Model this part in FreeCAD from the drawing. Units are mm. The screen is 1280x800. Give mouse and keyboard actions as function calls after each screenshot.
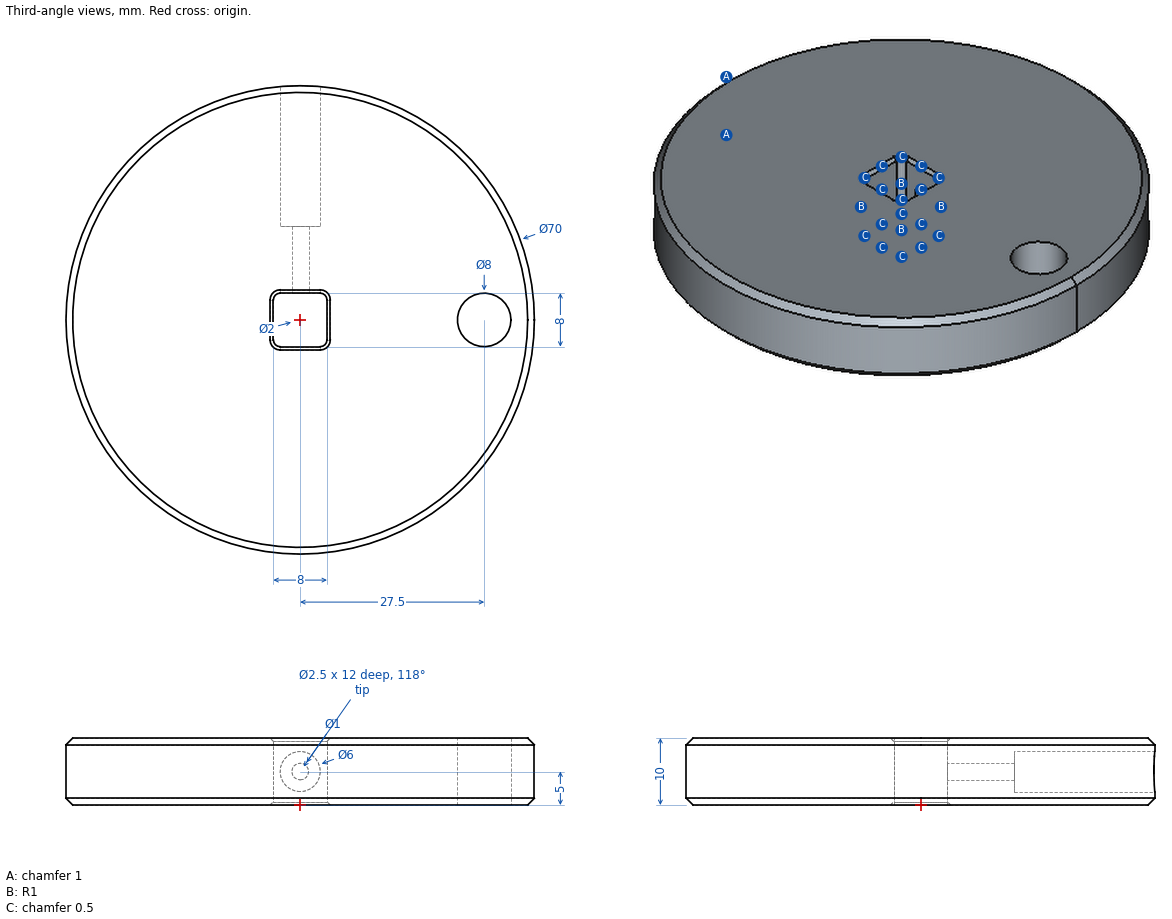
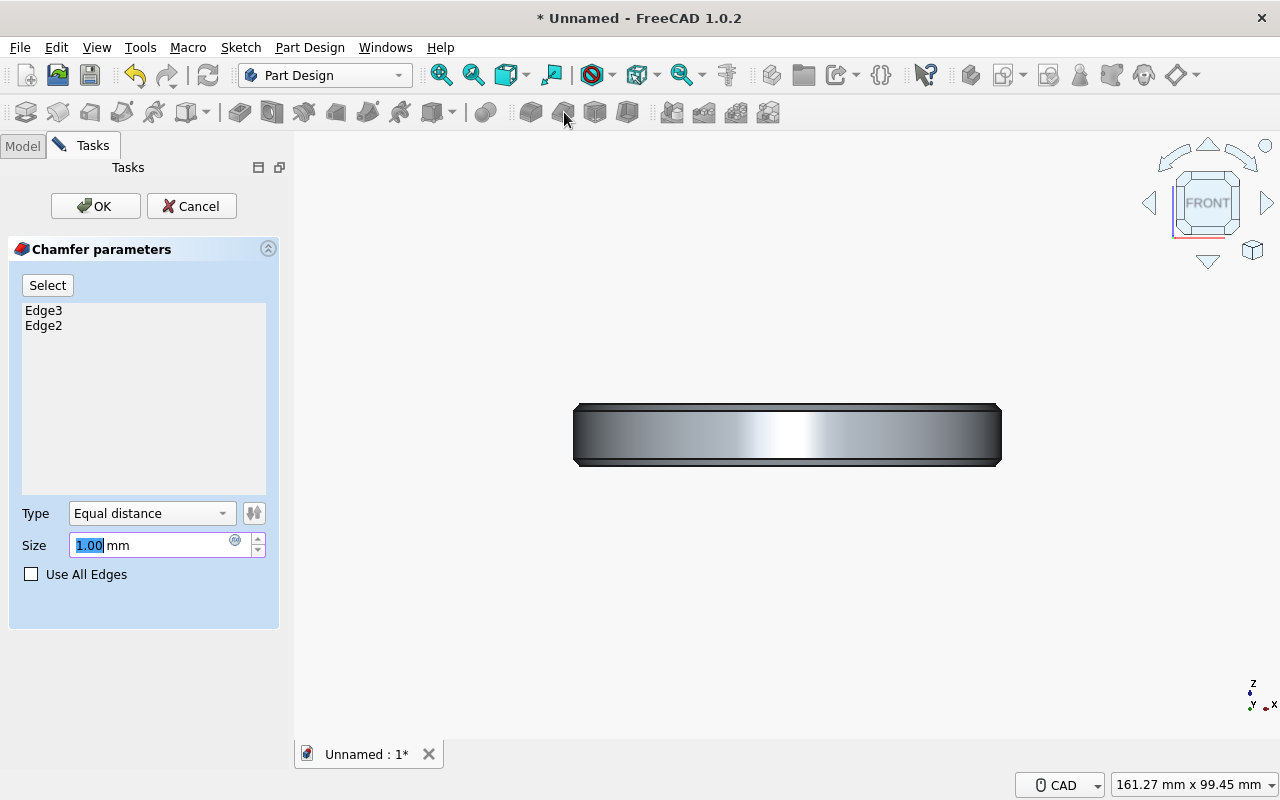
text(1)
key(Tab)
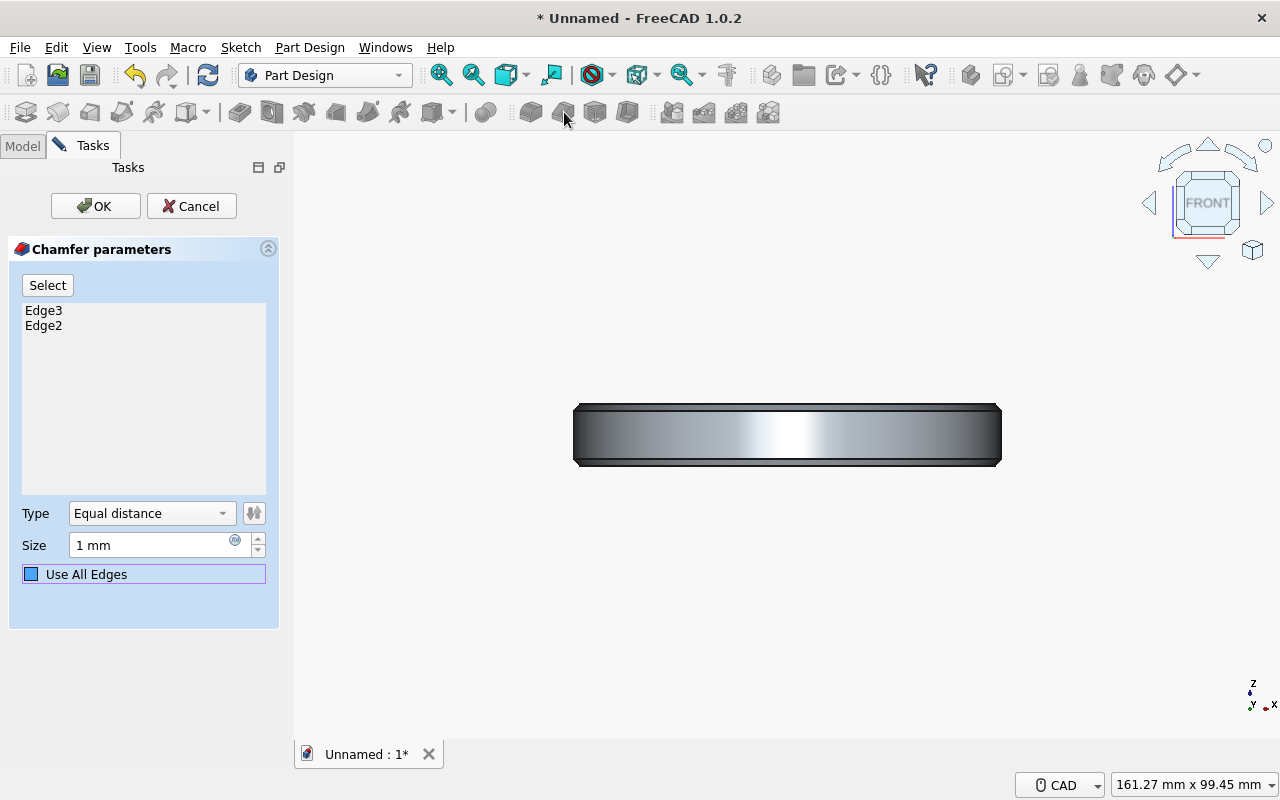
click(96, 206)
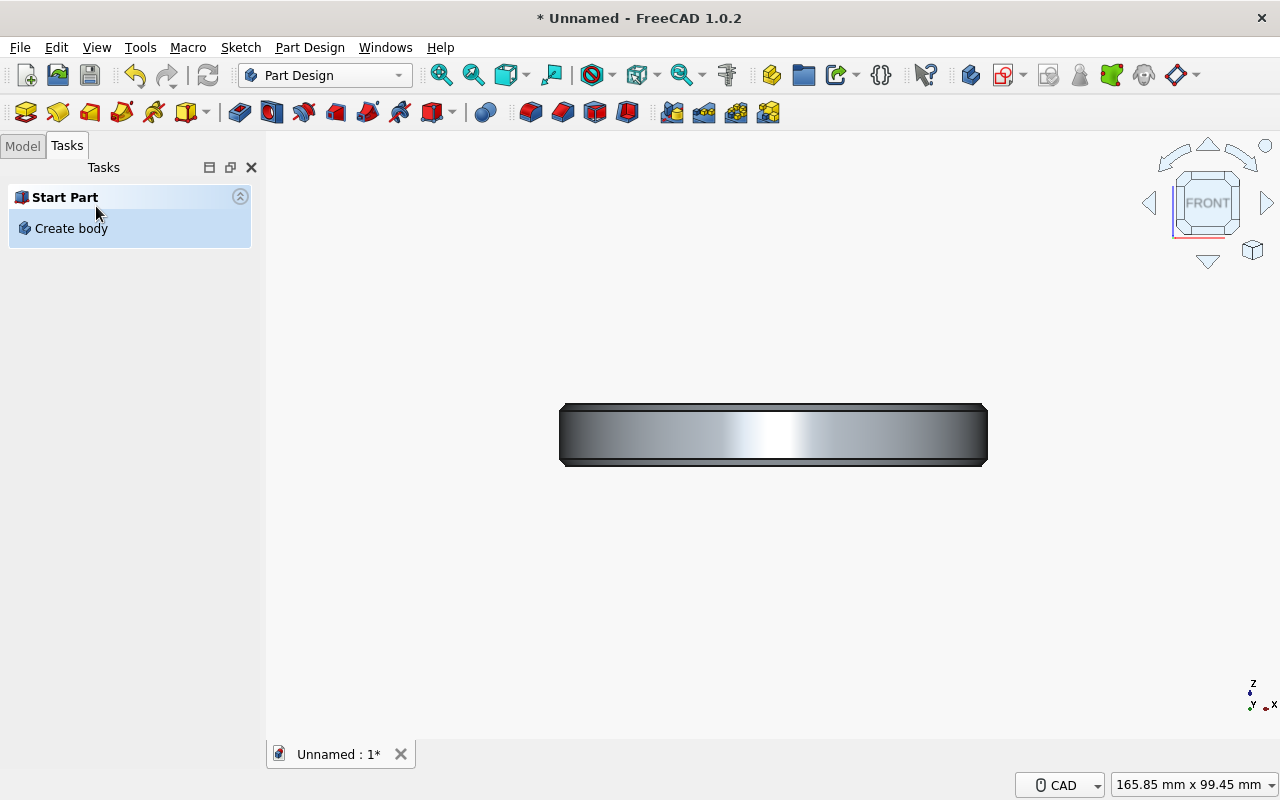
click(442, 76)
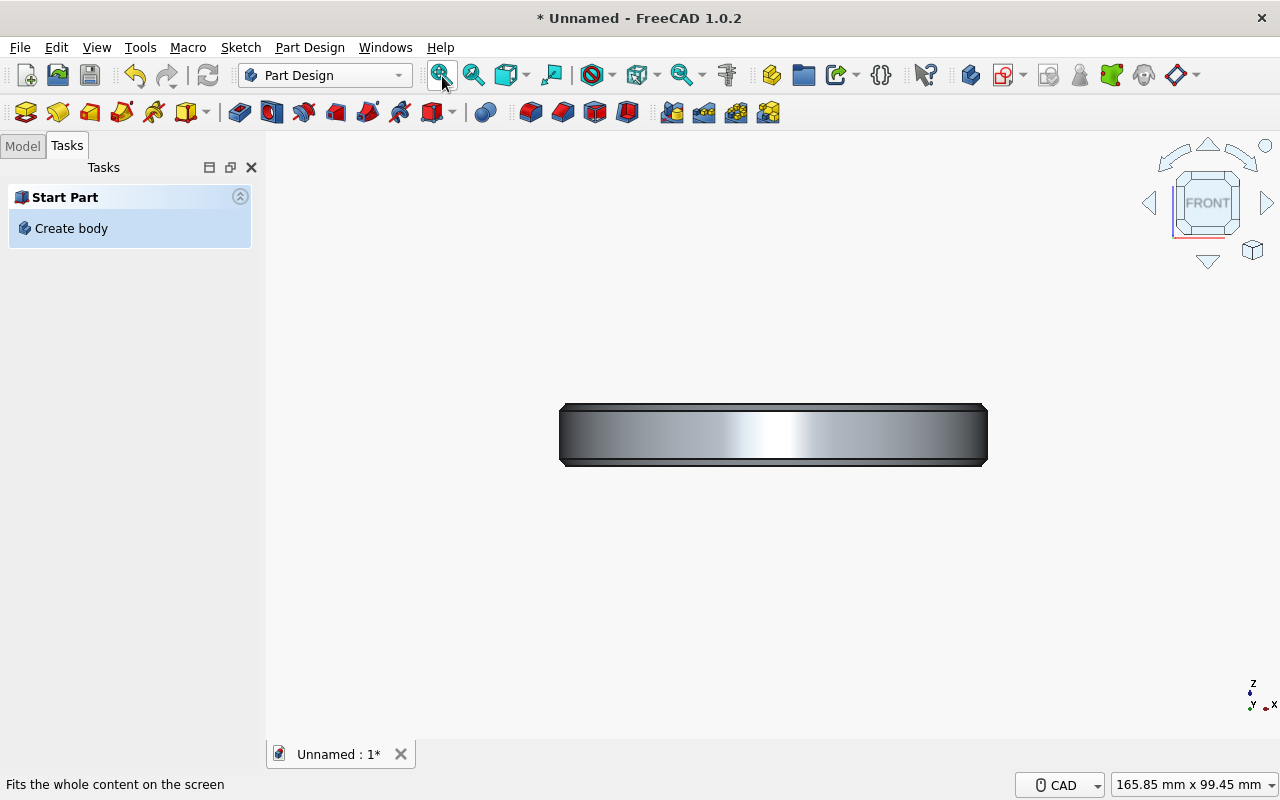
key(0)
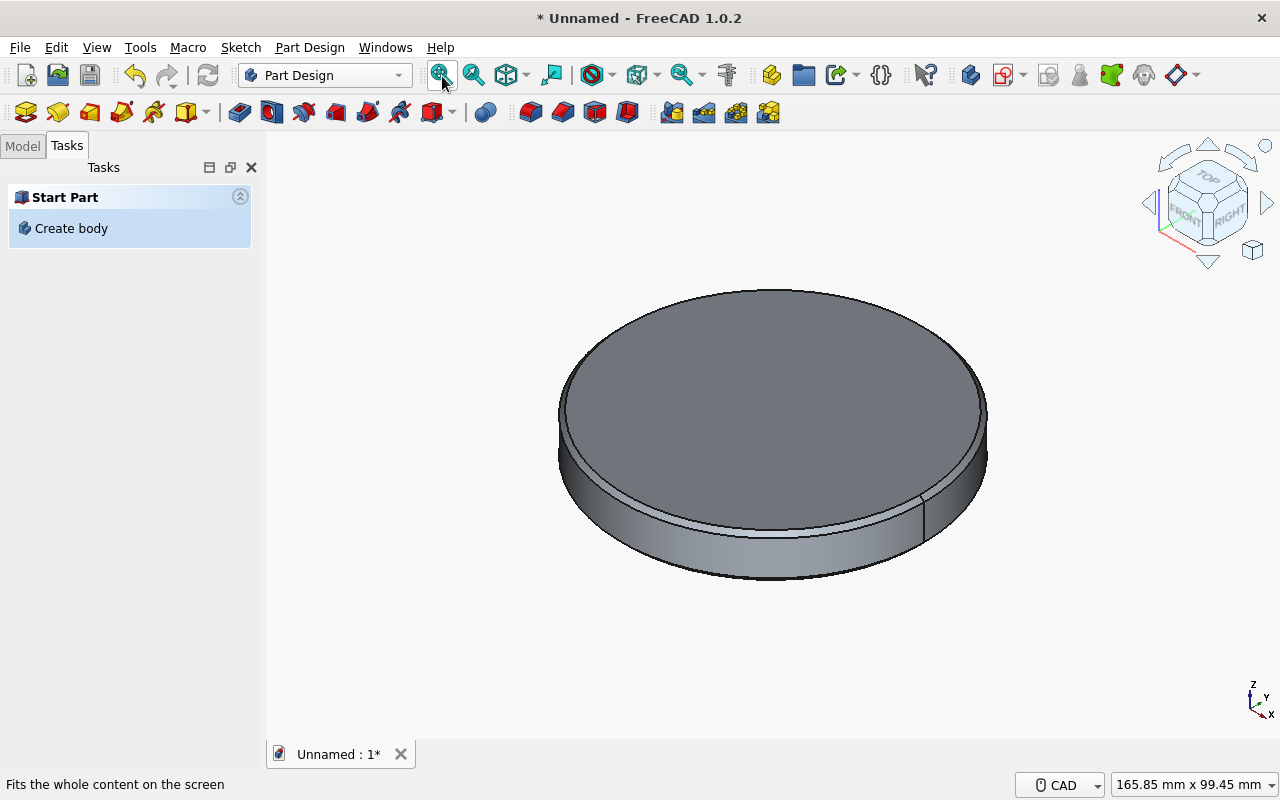
click(773, 409)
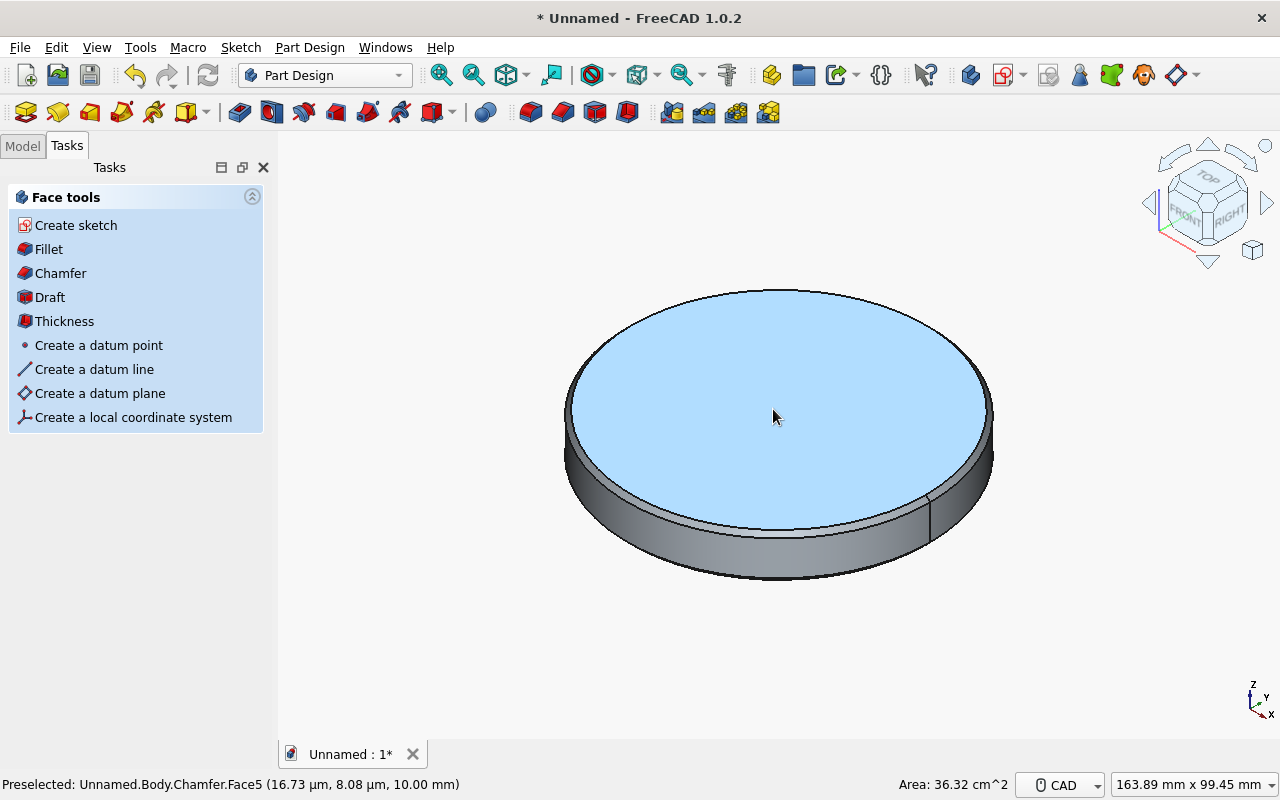
click(1004, 76)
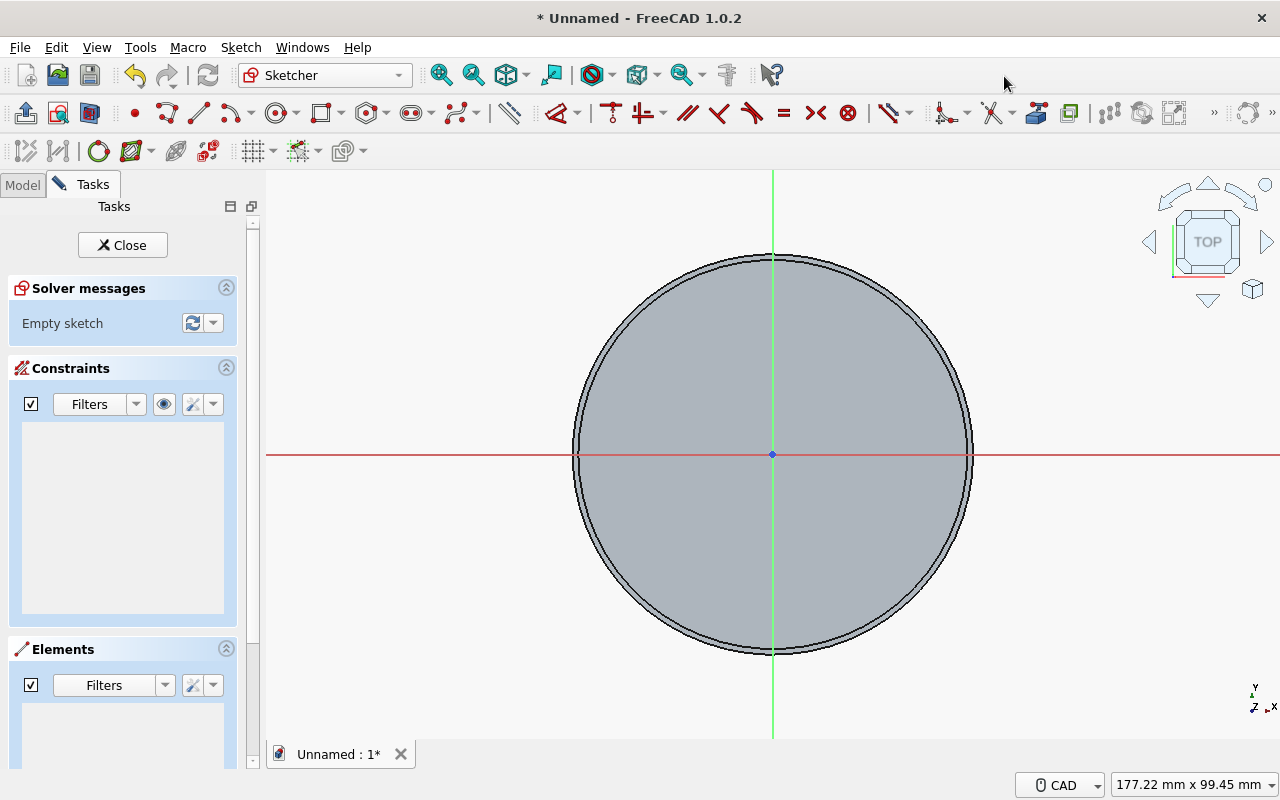
scroll(776, 455, up, 15)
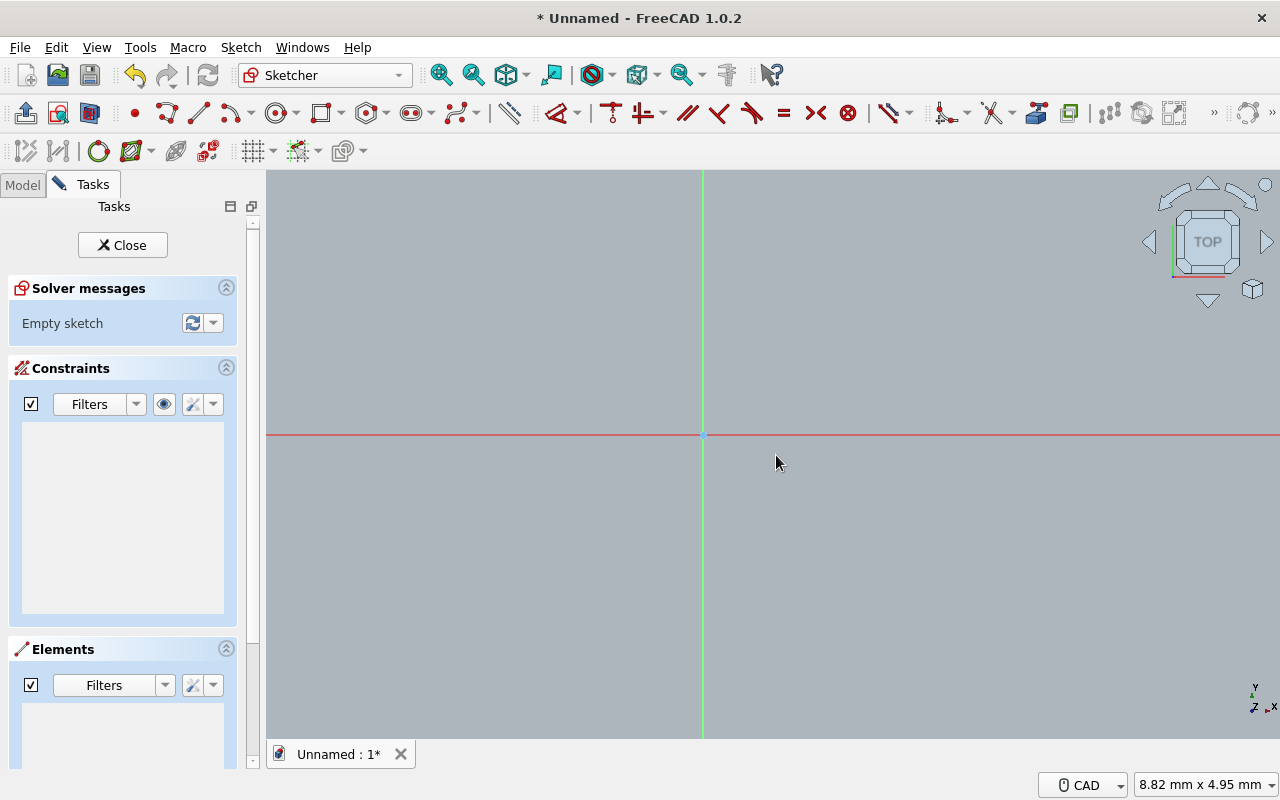
scroll(701, 397, up, 2)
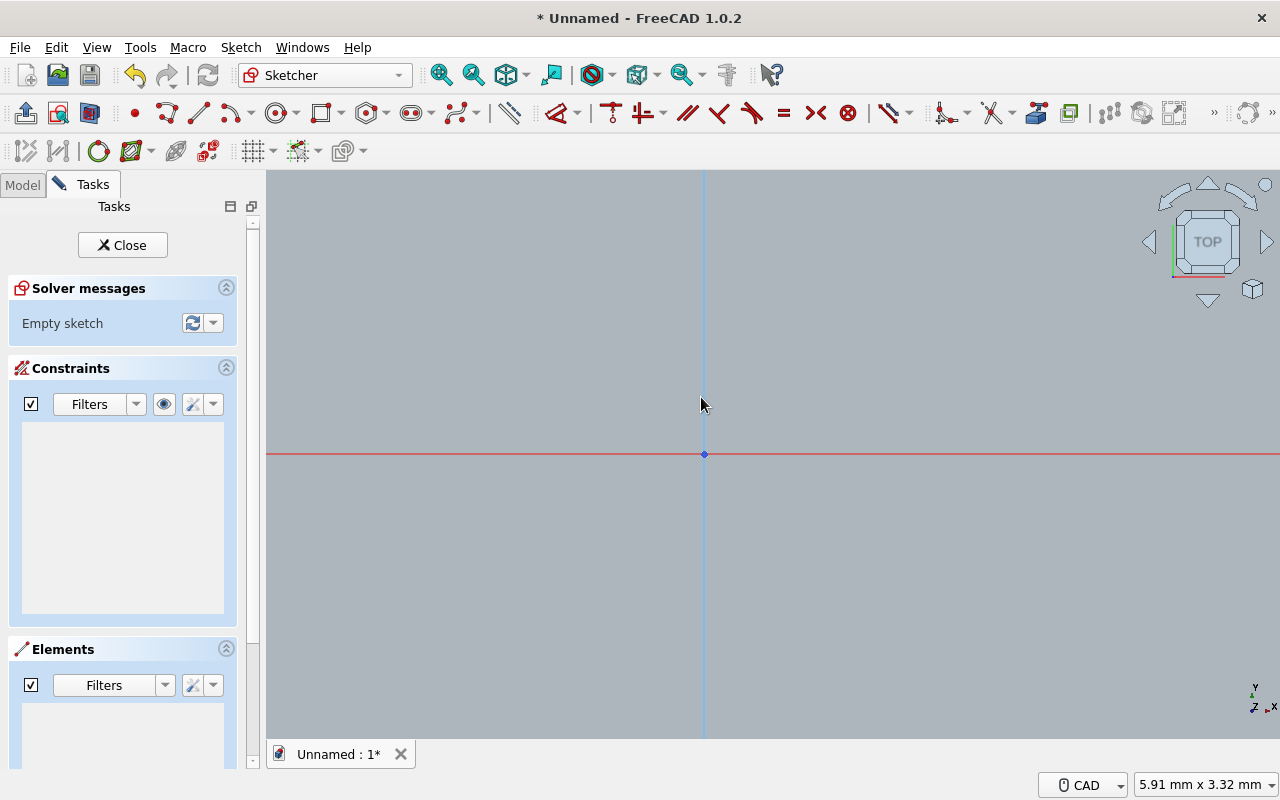
click(276, 114)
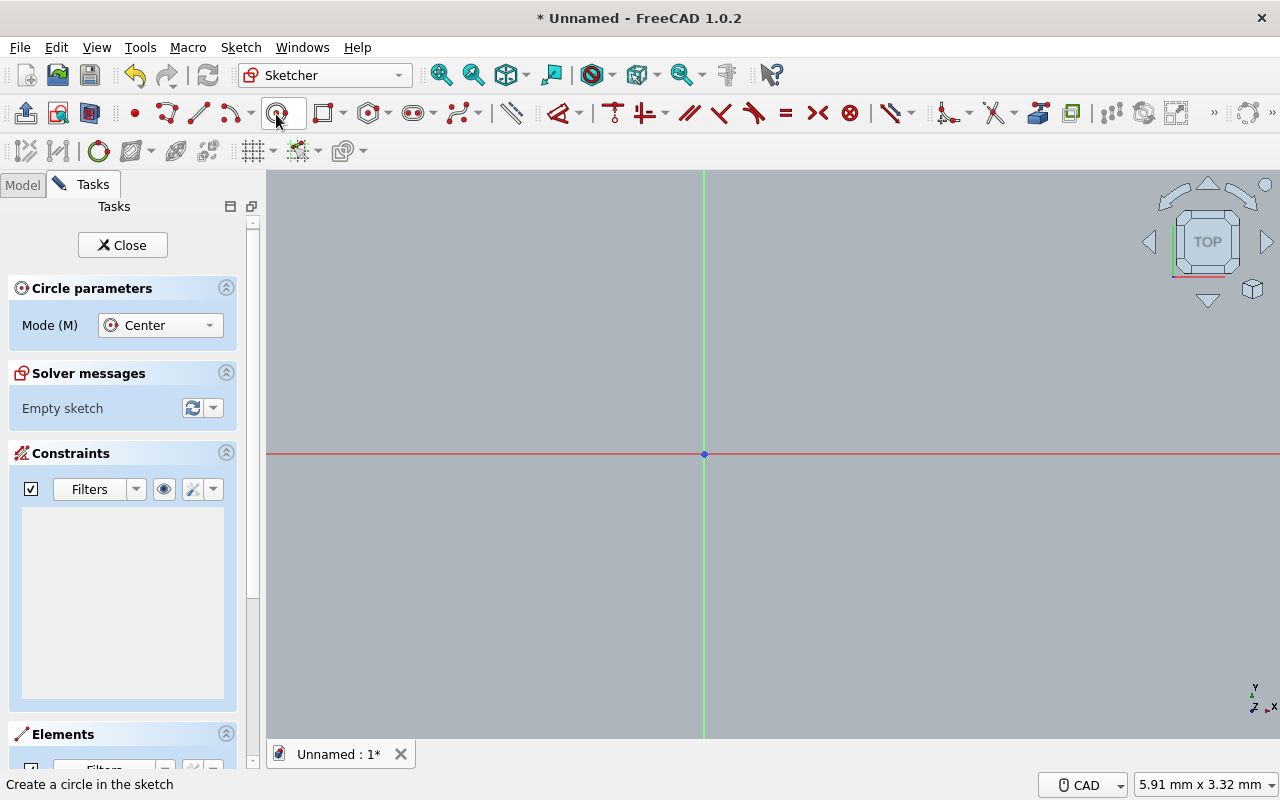
click(704, 454)
click(825, 333)
key(Escape)